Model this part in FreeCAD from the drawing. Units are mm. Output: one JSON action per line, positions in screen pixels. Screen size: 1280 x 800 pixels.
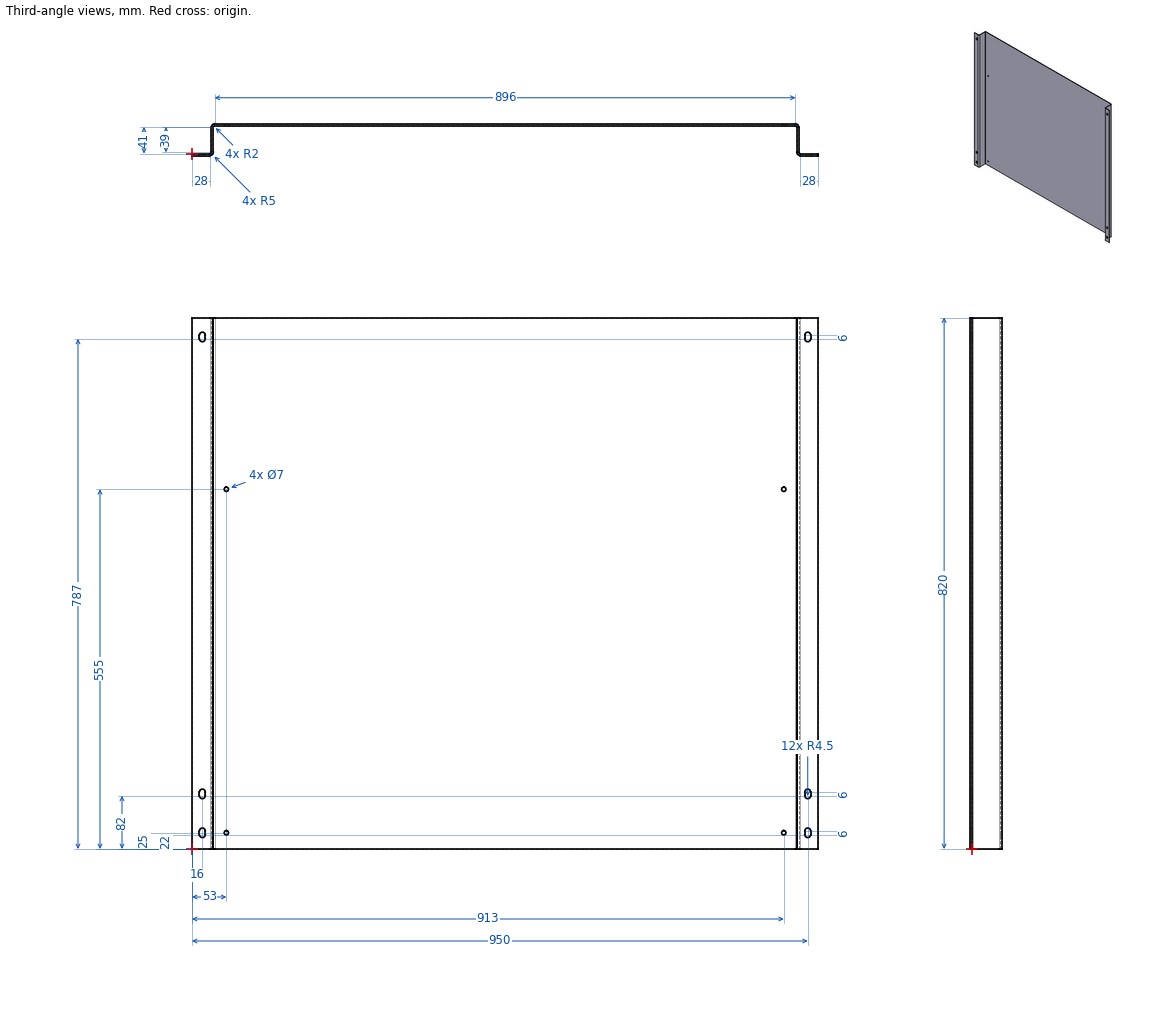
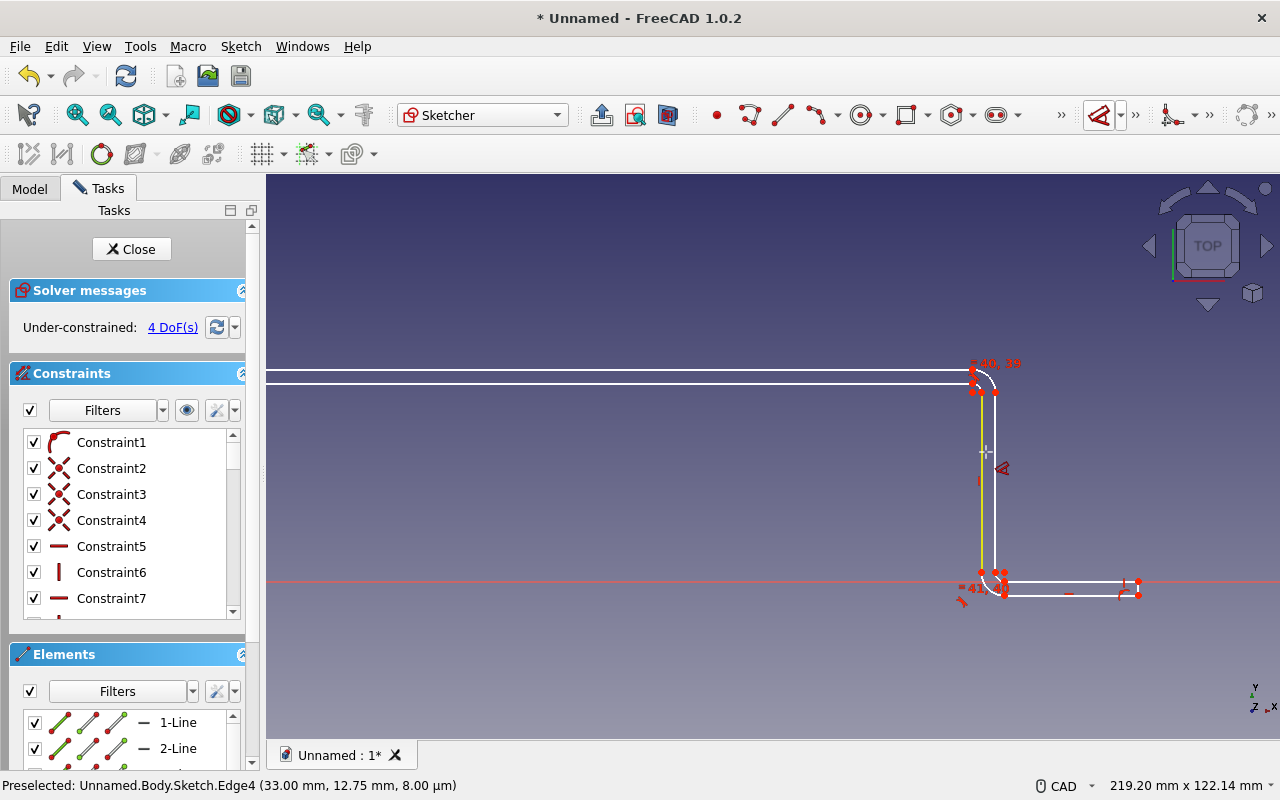
{"action": "left_click", "coordinate": [982, 447]}
{"action": "left_click", "coordinate": [1016, 483]}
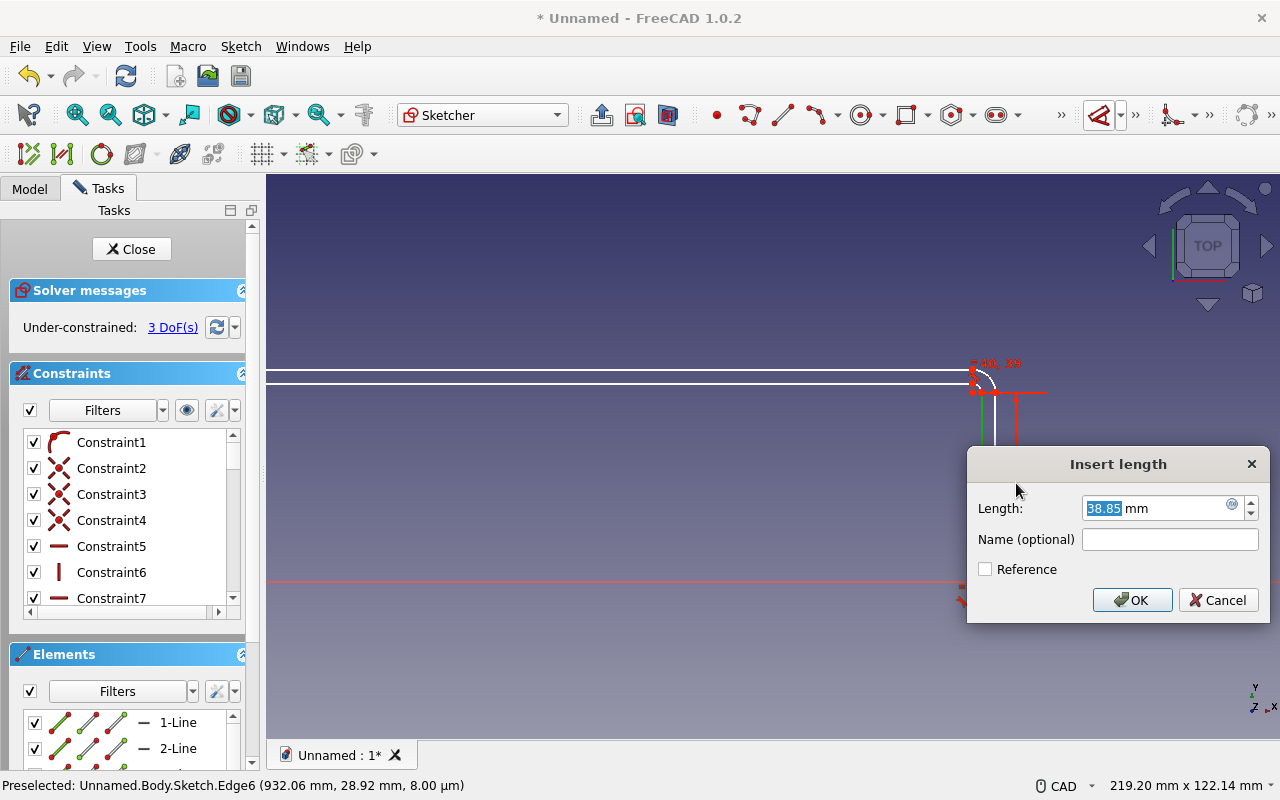
{"action": "type", "text": "39"}
{"action": "key", "text": "Return"}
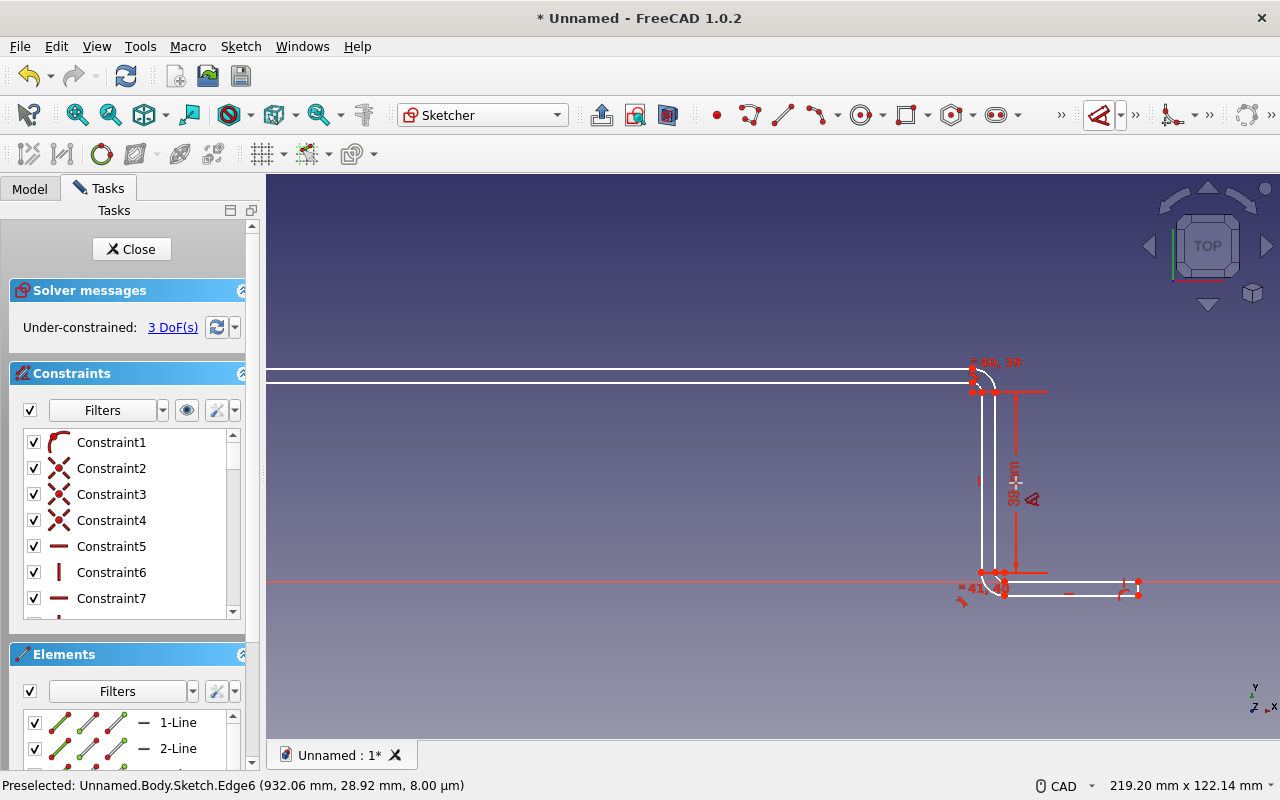
{"action": "left_click", "coordinate": [1045, 596]}
{"action": "left_click", "coordinate": [1060, 630]}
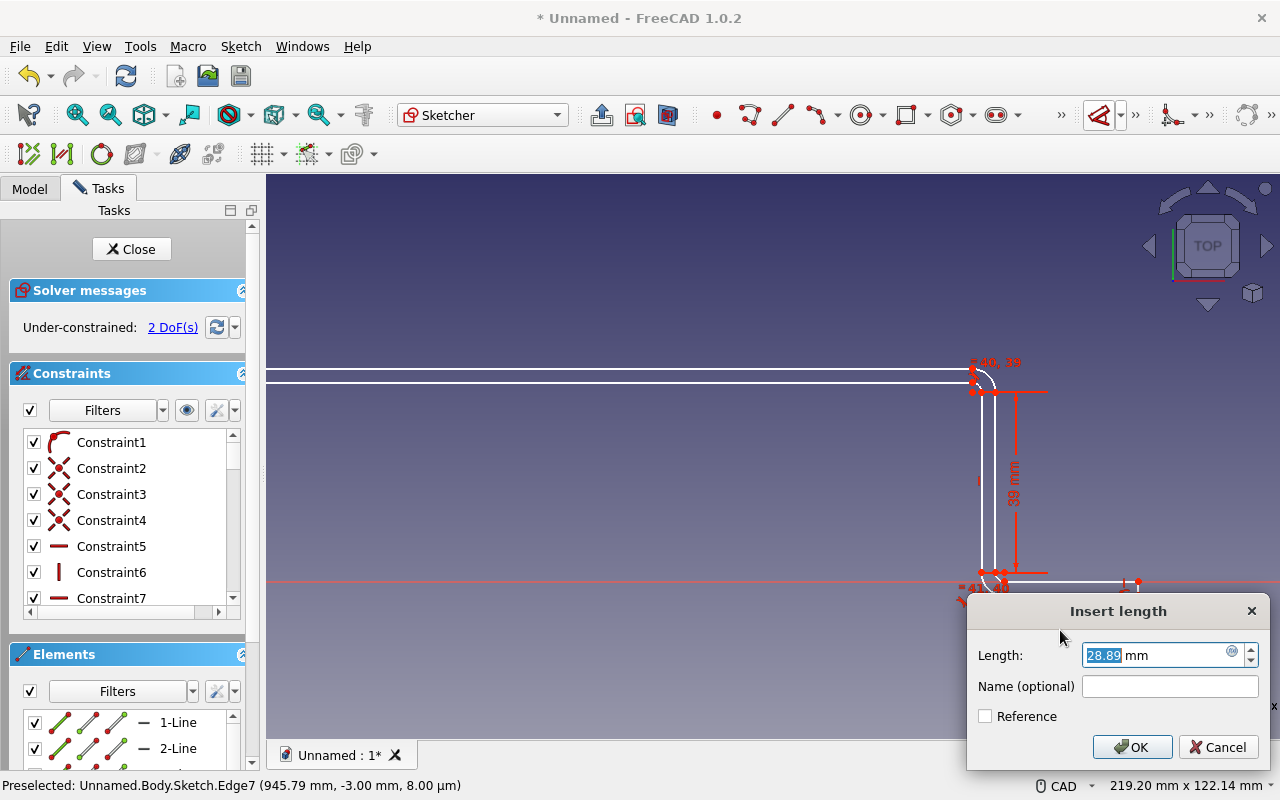
{"action": "type", "text": "28"}
{"action": "key", "text": "Return"}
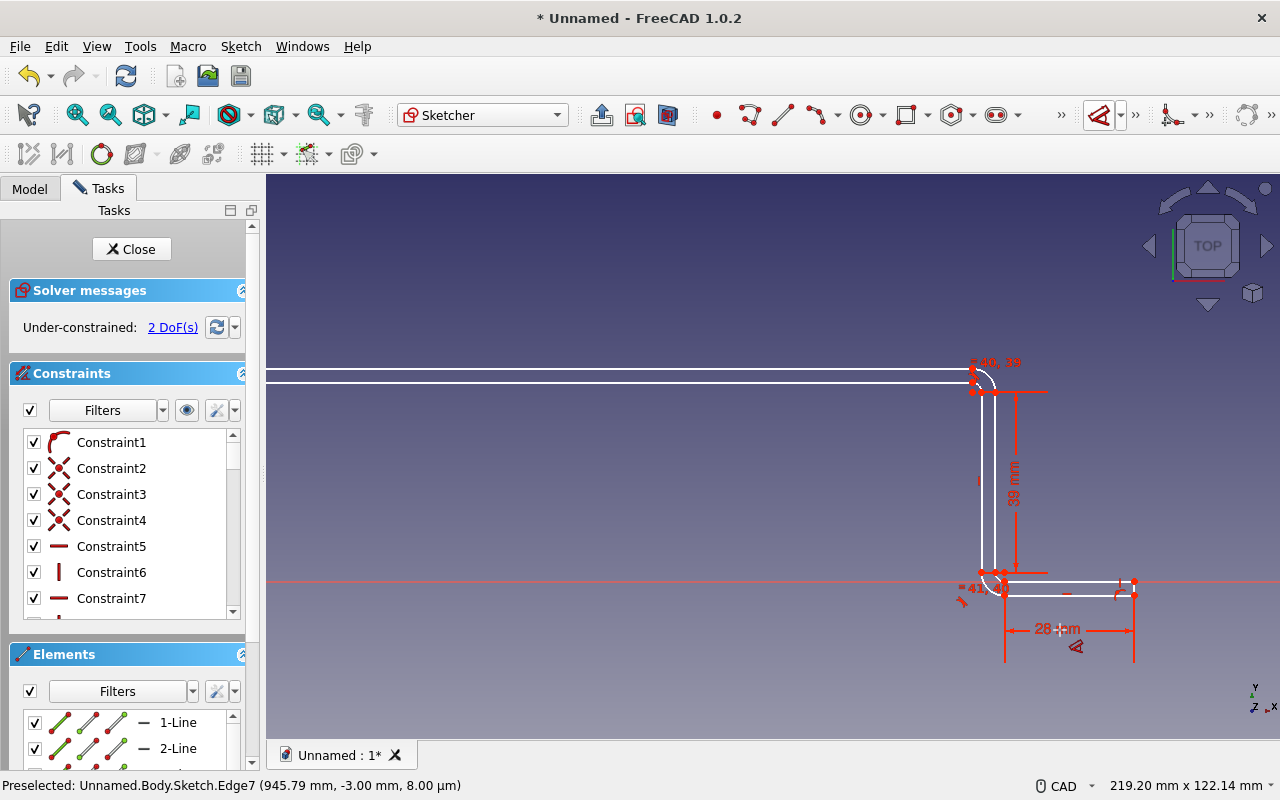
{"action": "scroll", "coordinate": [986, 452], "scroll_direction": "down", "scroll_amount": 10}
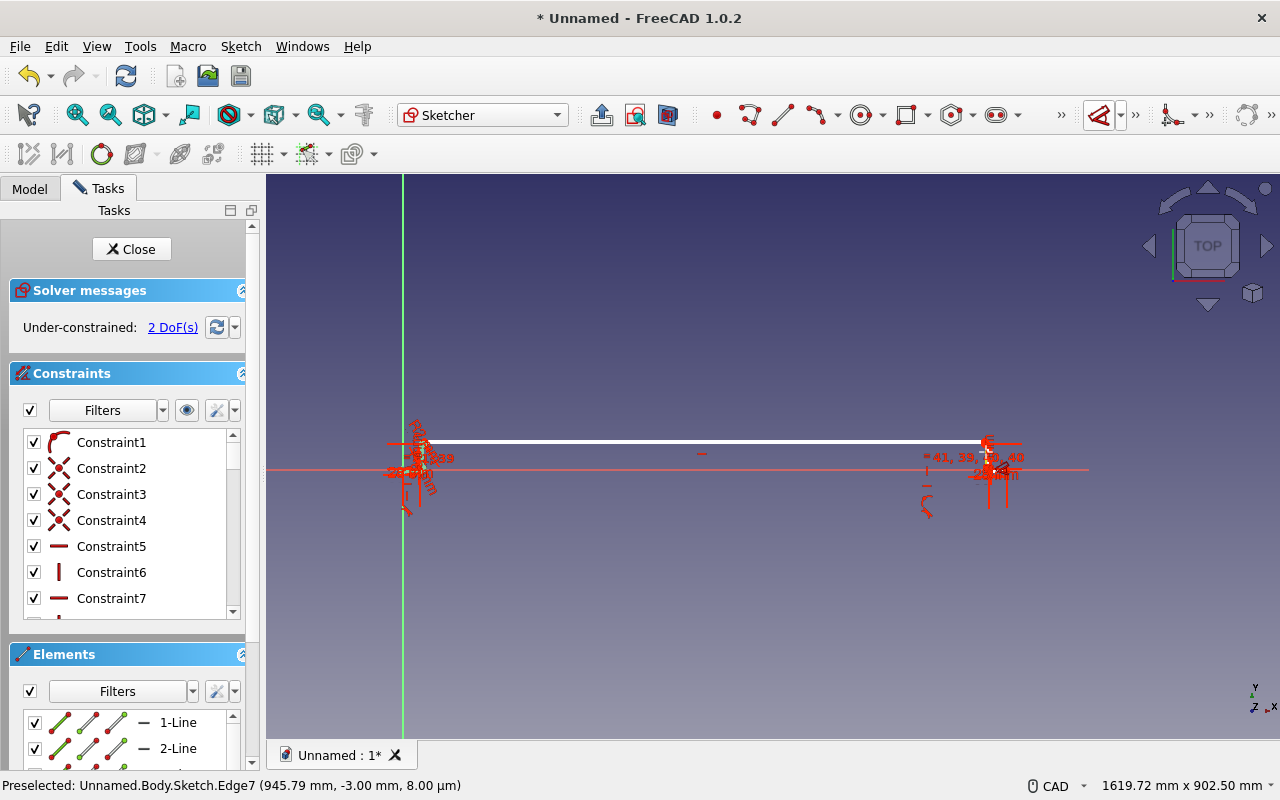
{"action": "scroll", "coordinate": [593, 443], "scroll_direction": "up", "scroll_amount": 10}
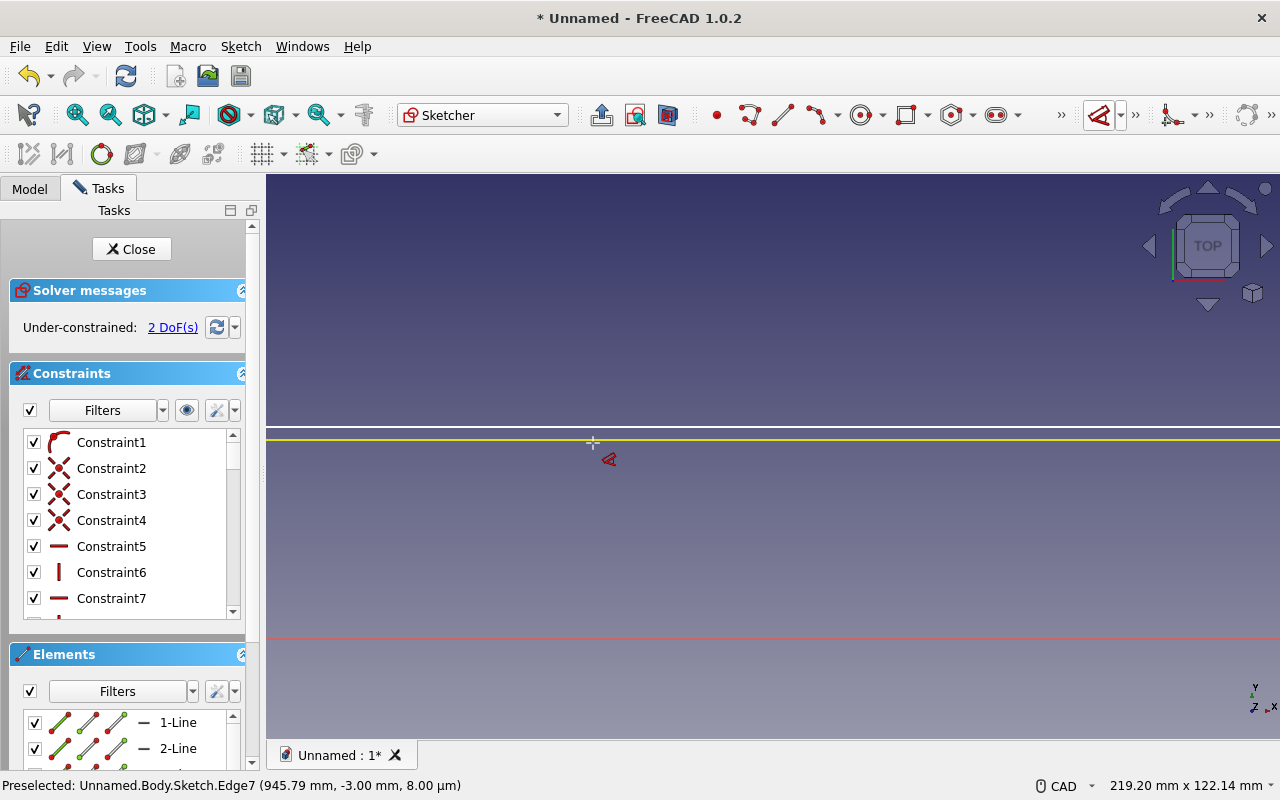
{"action": "left_click", "coordinate": [587, 440]}
{"action": "left_click", "coordinate": [704, 406]}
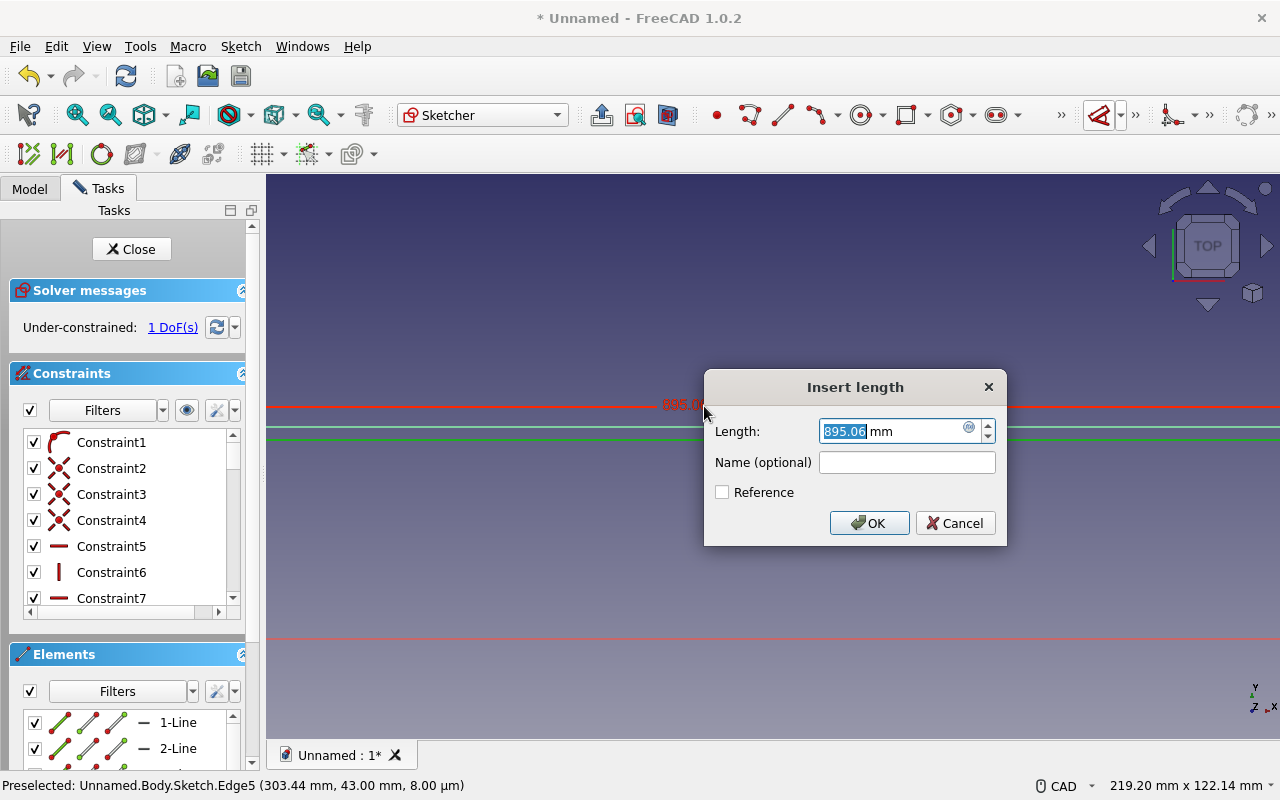
{"action": "type", "text": "896"}
{"action": "key", "text": "Return"}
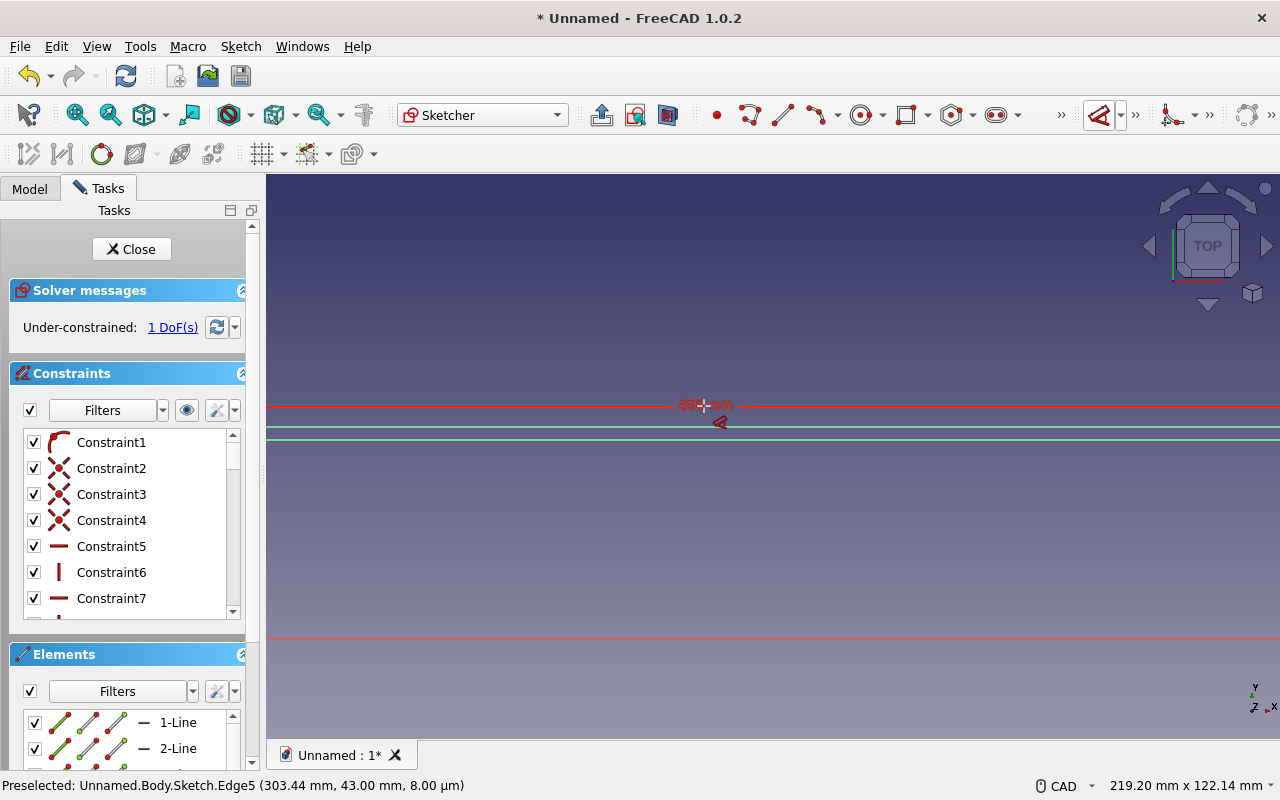
{"action": "scroll", "coordinate": [593, 443], "scroll_direction": "down", "scroll_amount": 10}